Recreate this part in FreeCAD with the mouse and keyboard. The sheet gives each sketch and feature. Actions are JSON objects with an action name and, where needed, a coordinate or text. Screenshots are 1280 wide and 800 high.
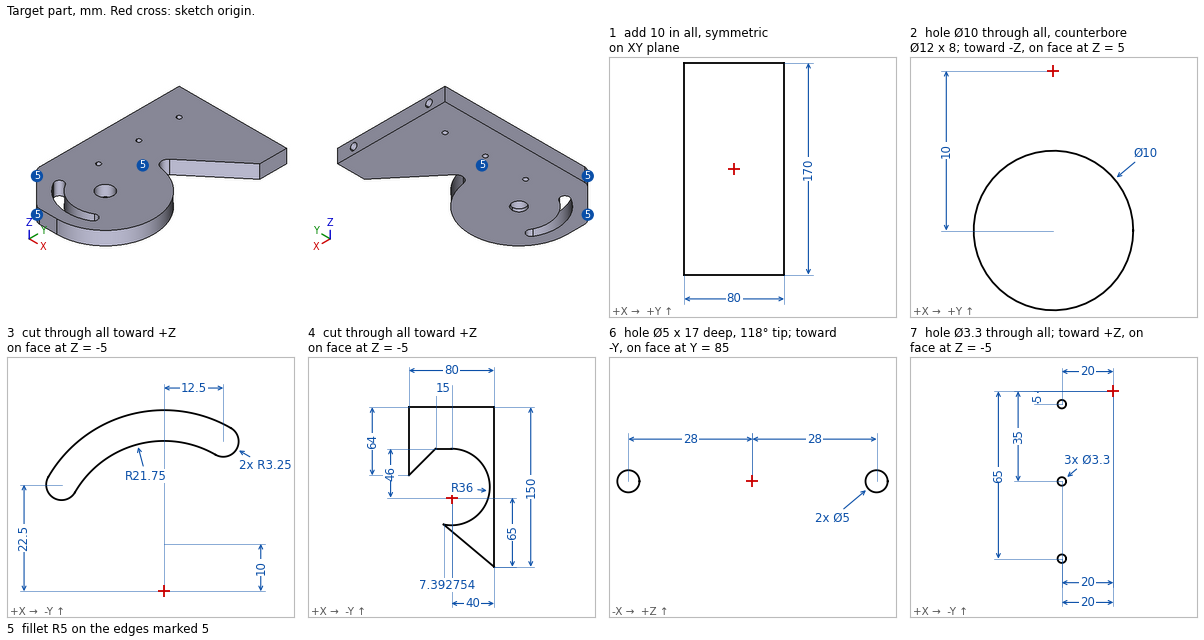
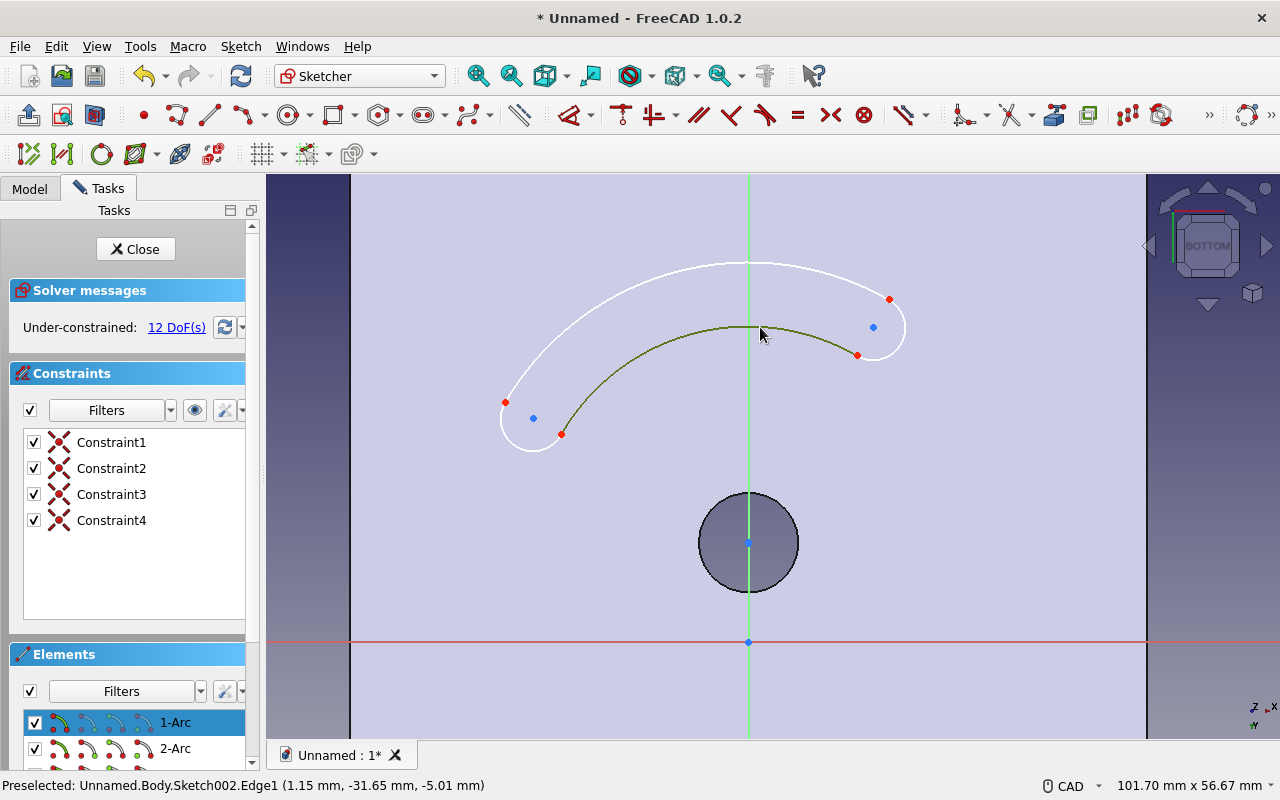
{"action": "left_click", "coordinate": [886, 357]}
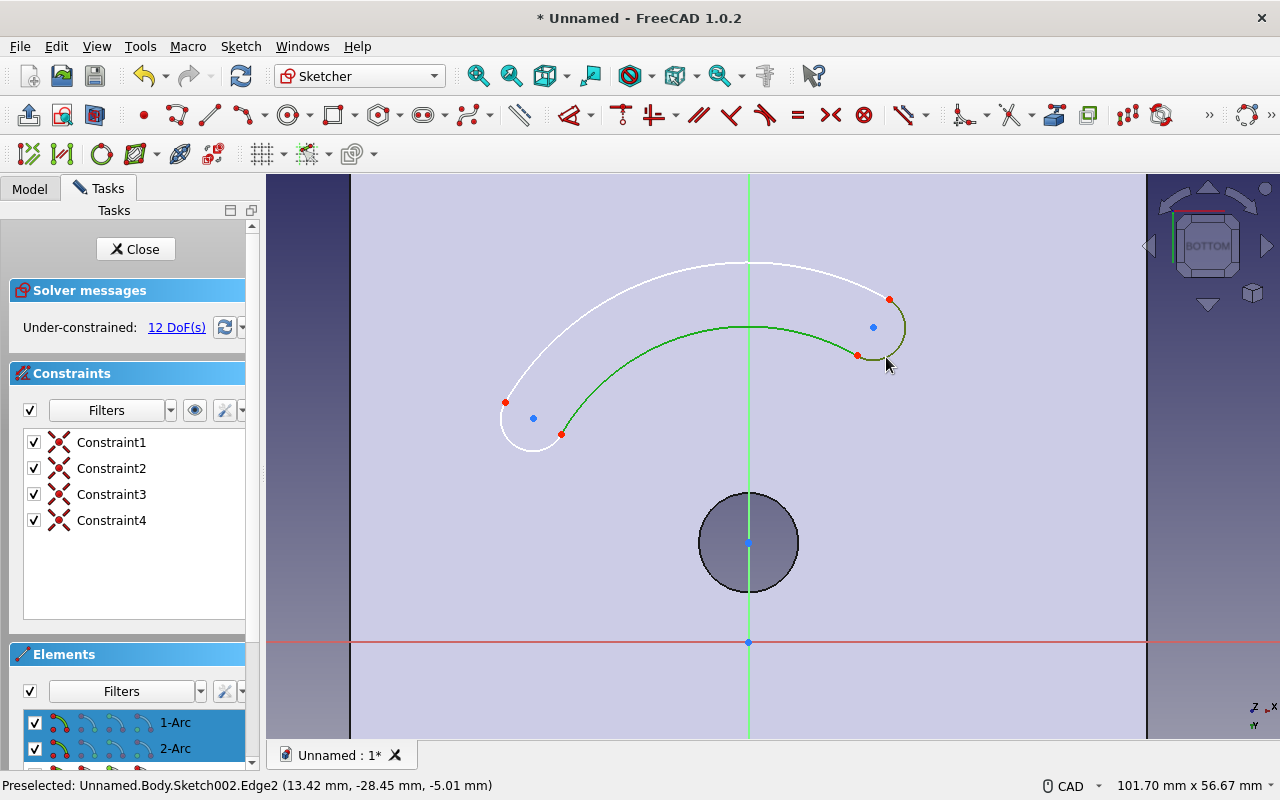
{"action": "key", "text": "t"}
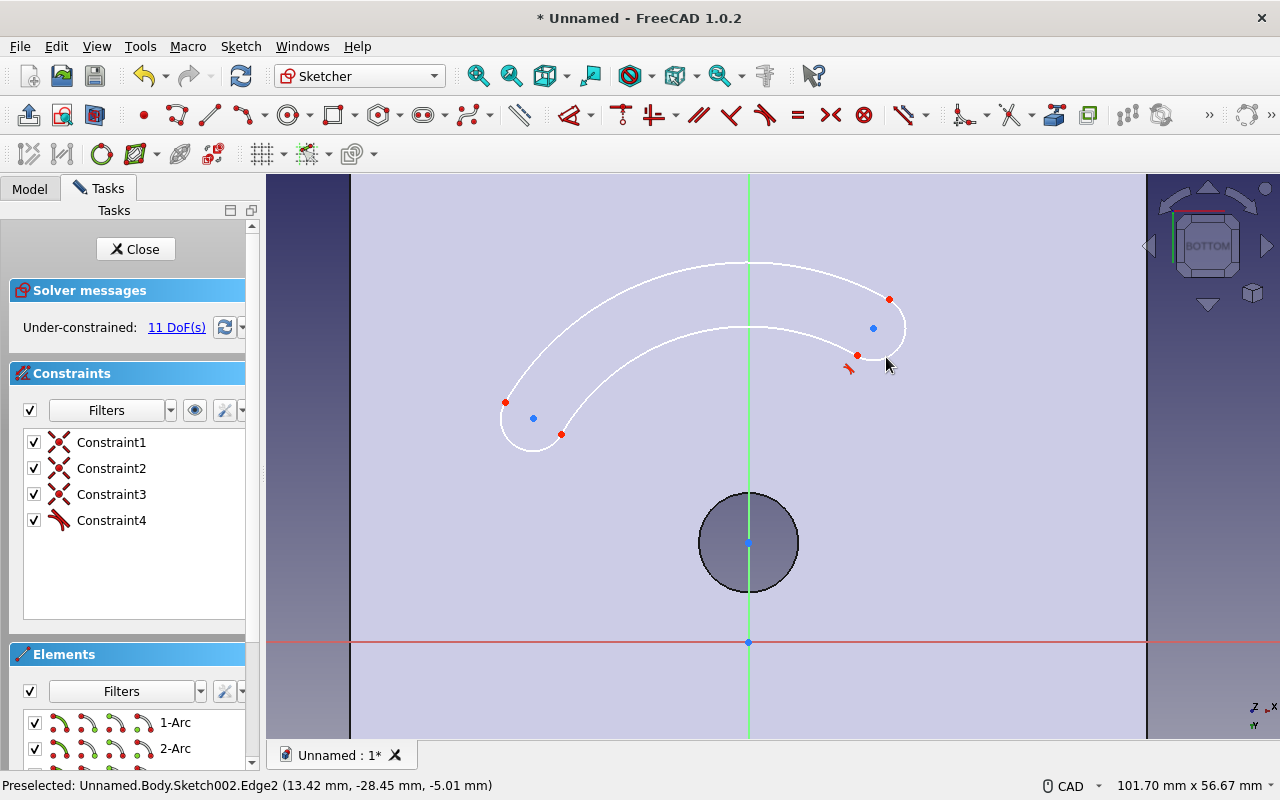
{"action": "left_click", "coordinate": [760, 327]}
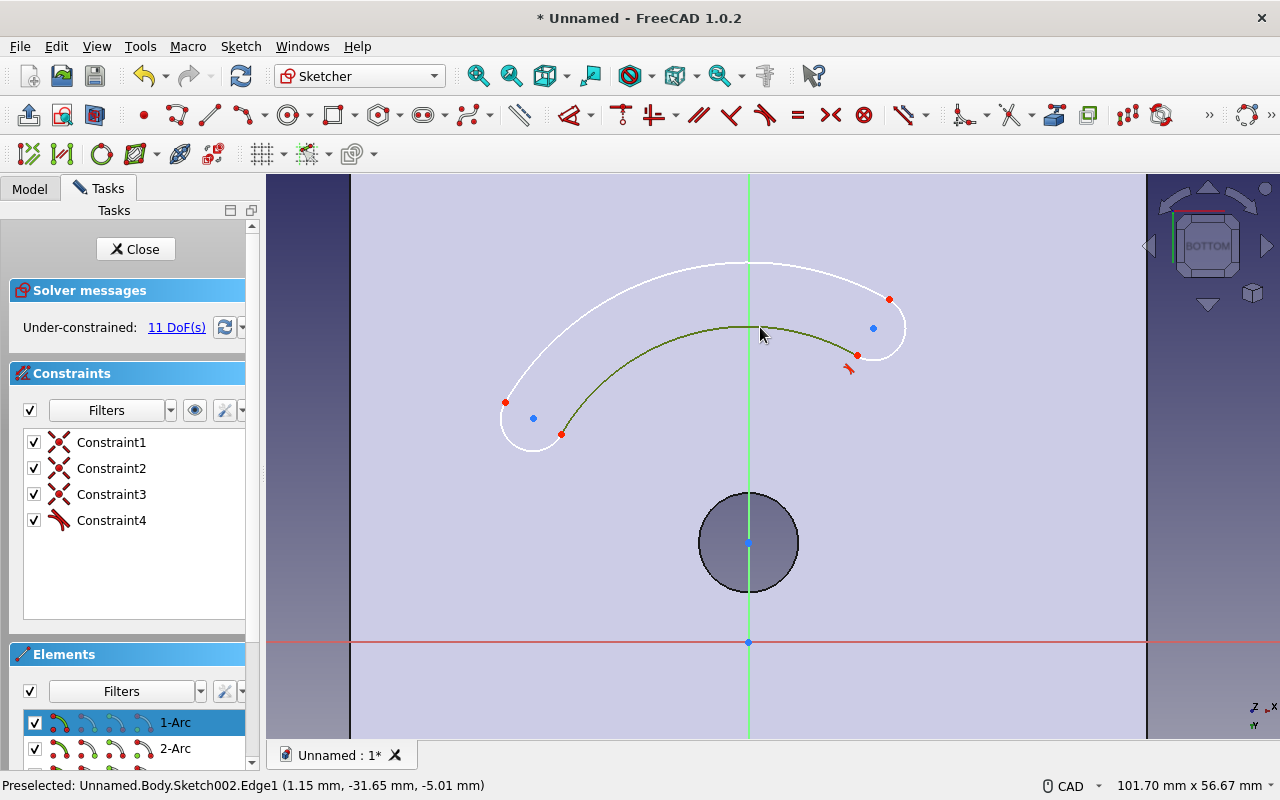
{"action": "left_click", "coordinate": [504, 432]}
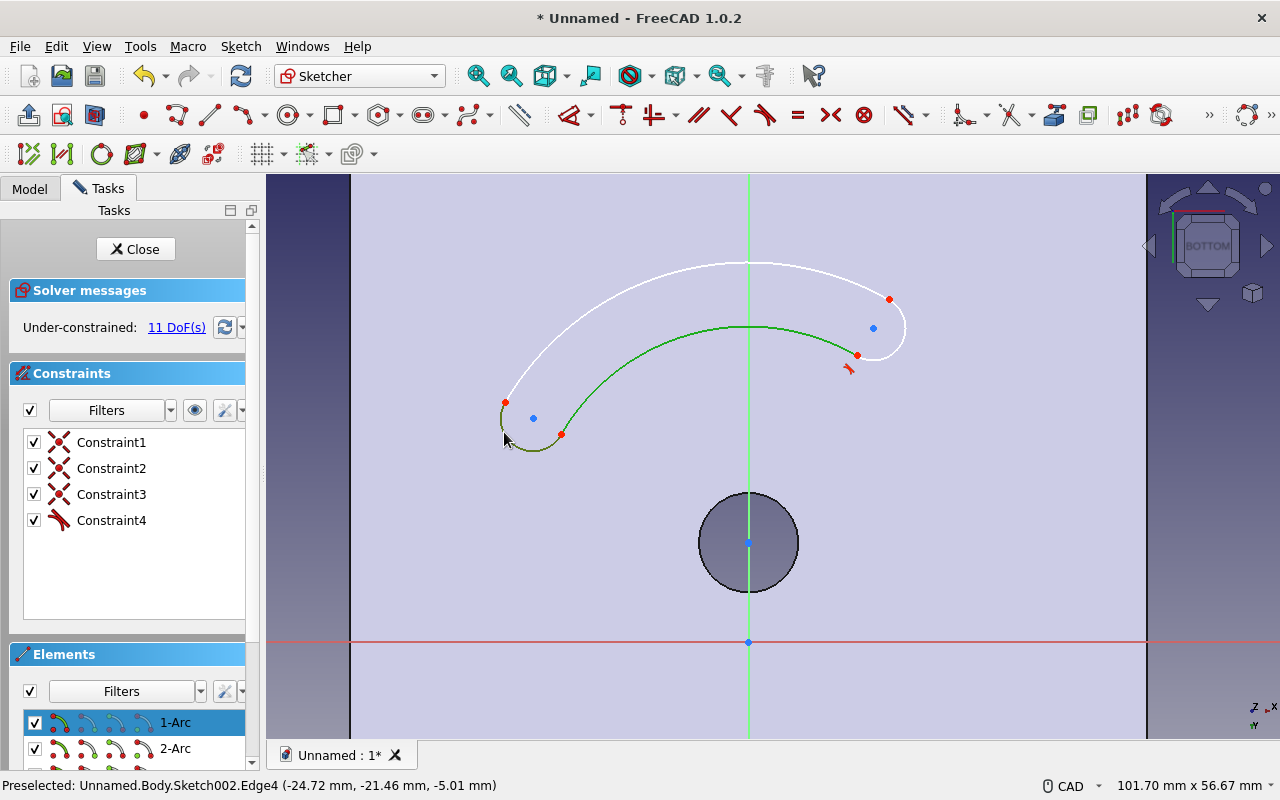
{"action": "key", "text": "t"}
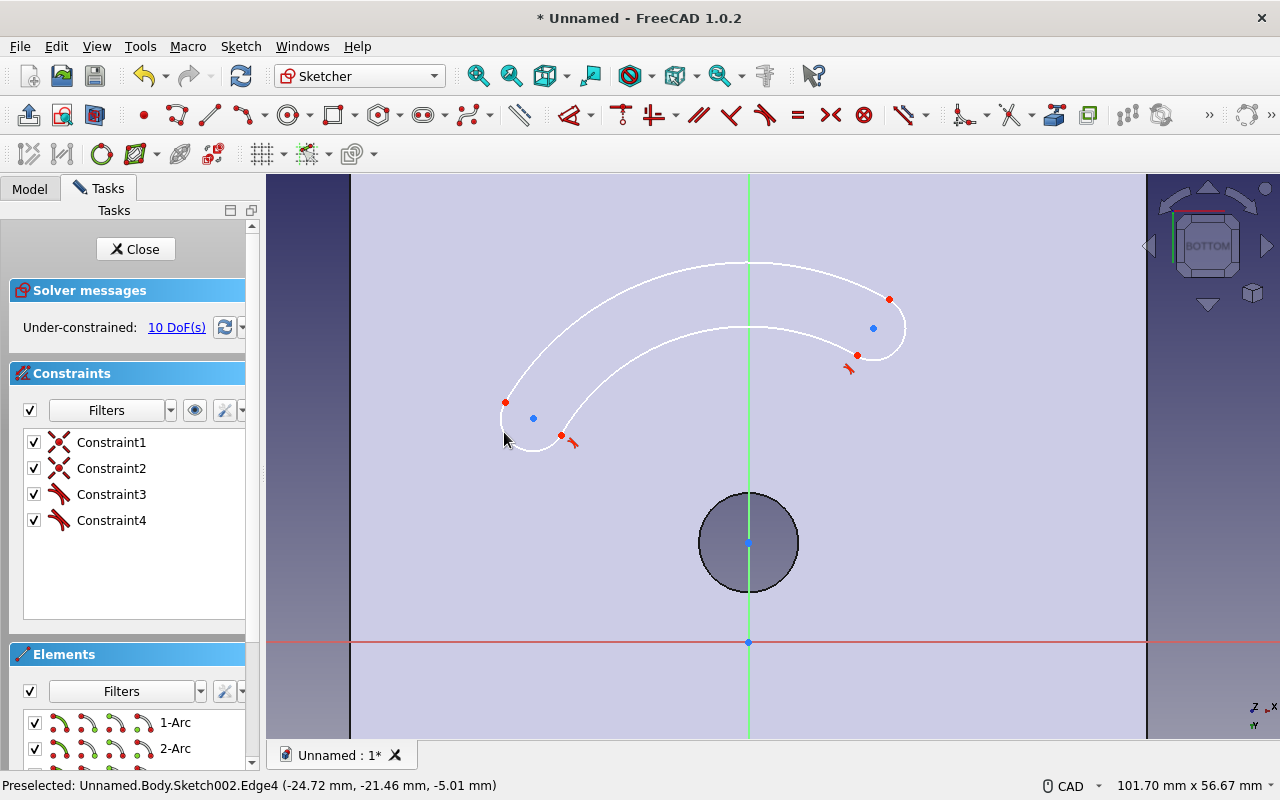
{"action": "left_click", "coordinate": [886, 358]}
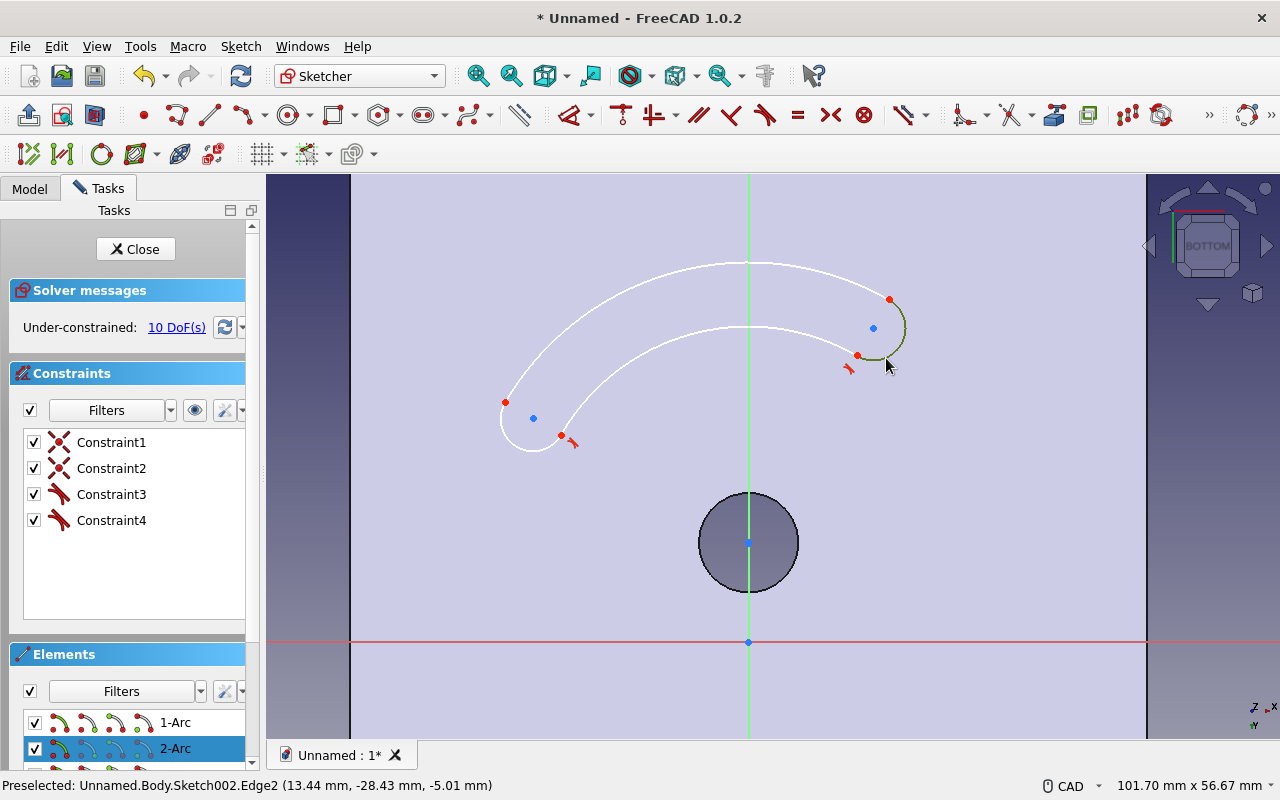
{"action": "left_click", "coordinate": [763, 263]}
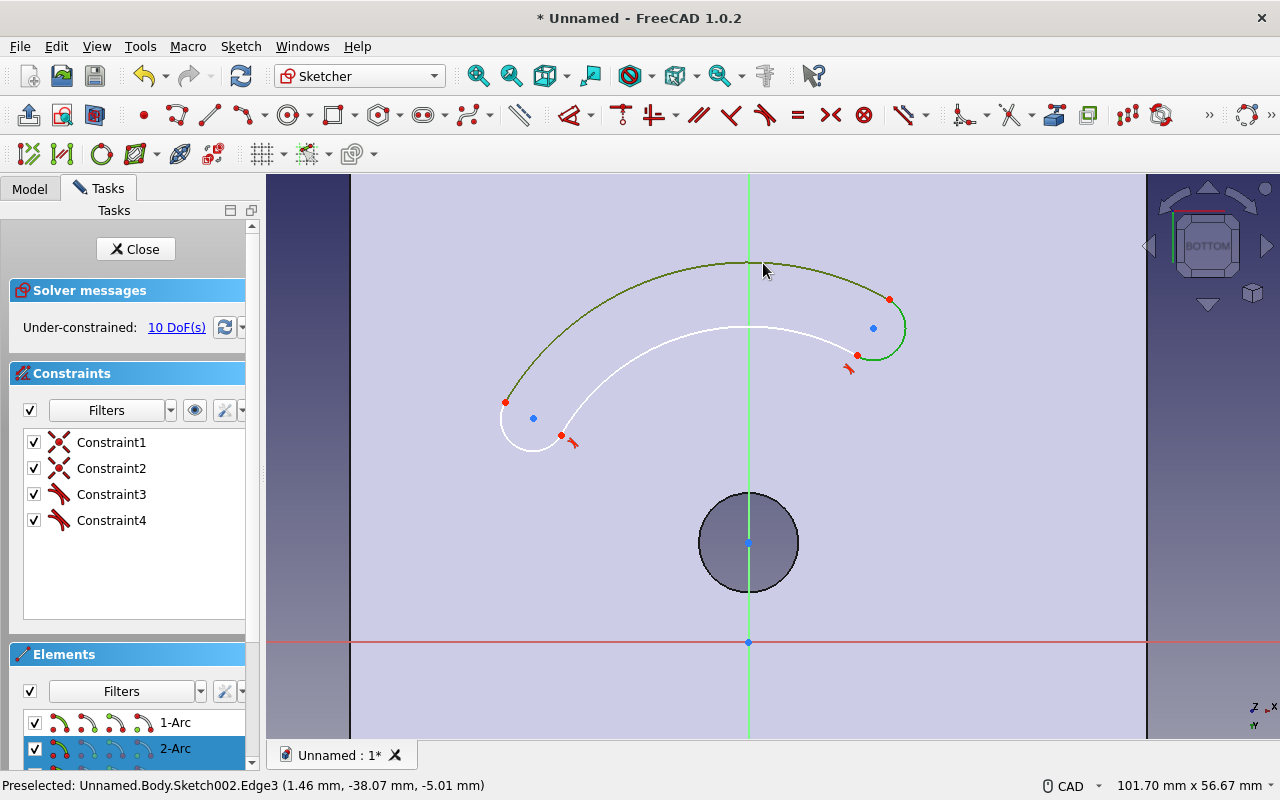
{"action": "key", "text": "t"}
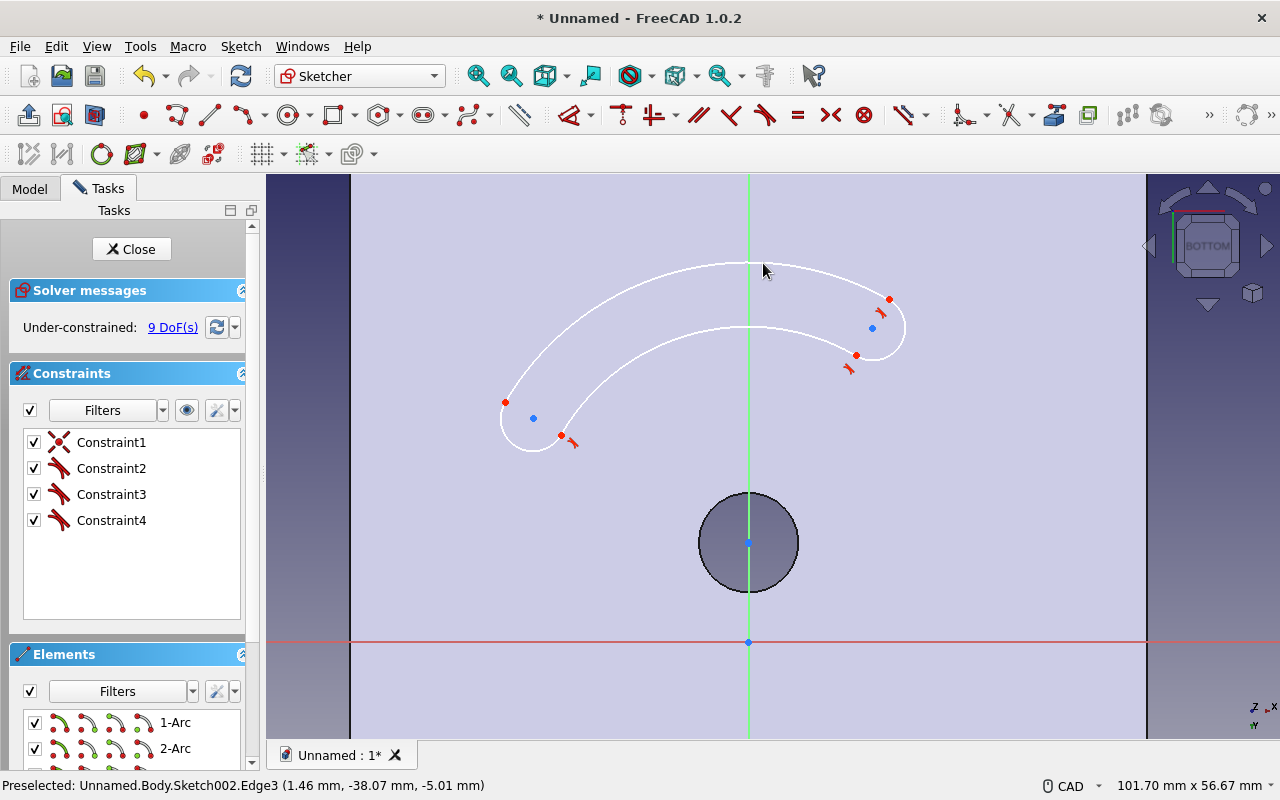
{"action": "left_click", "coordinate": [763, 263]}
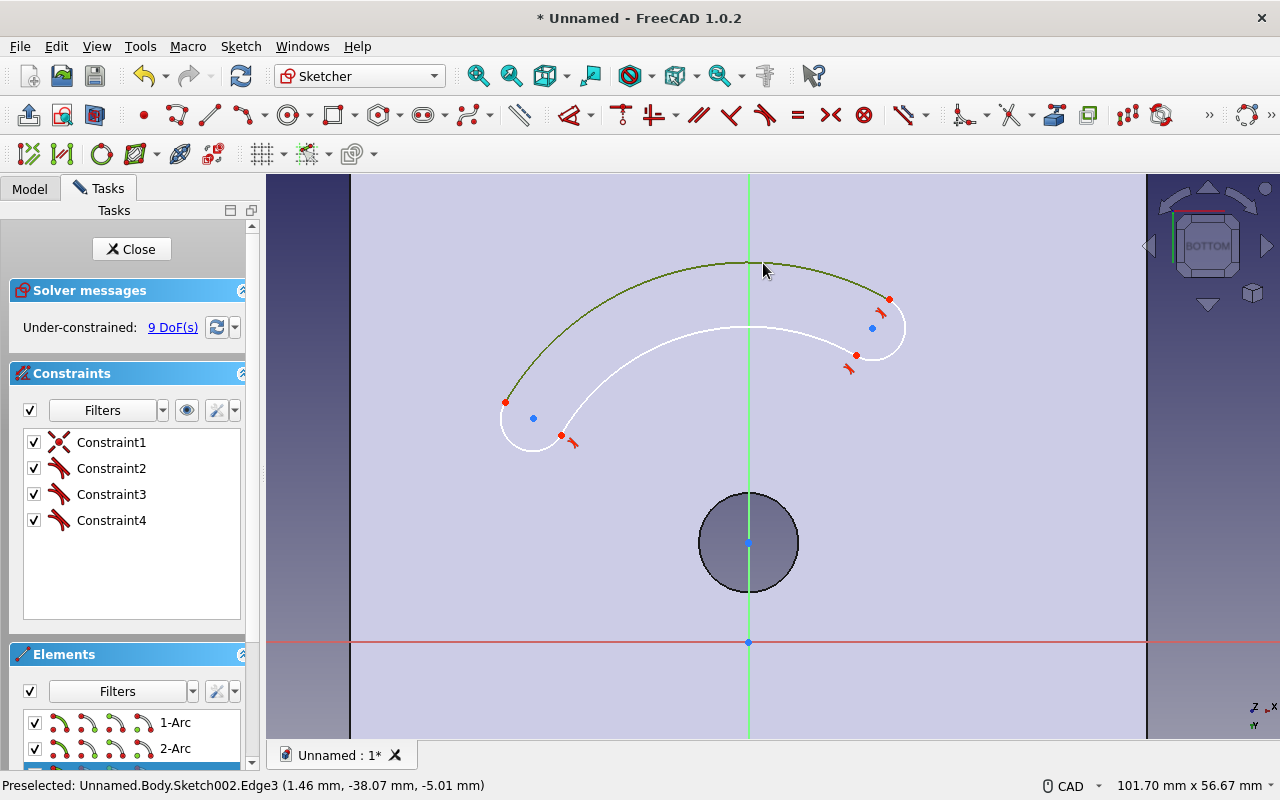
{"action": "left_click", "coordinate": [504, 432]}